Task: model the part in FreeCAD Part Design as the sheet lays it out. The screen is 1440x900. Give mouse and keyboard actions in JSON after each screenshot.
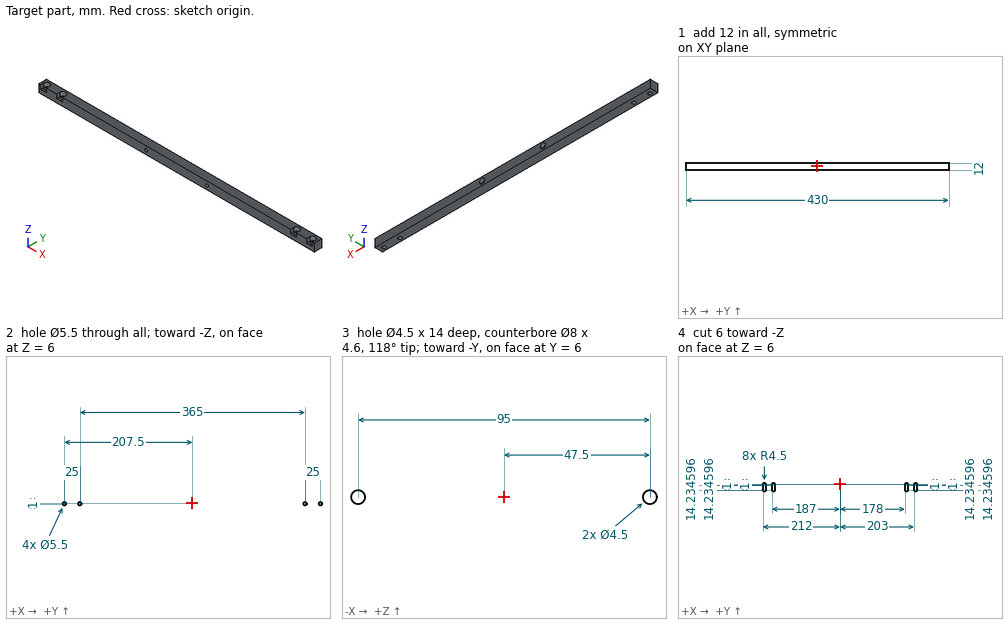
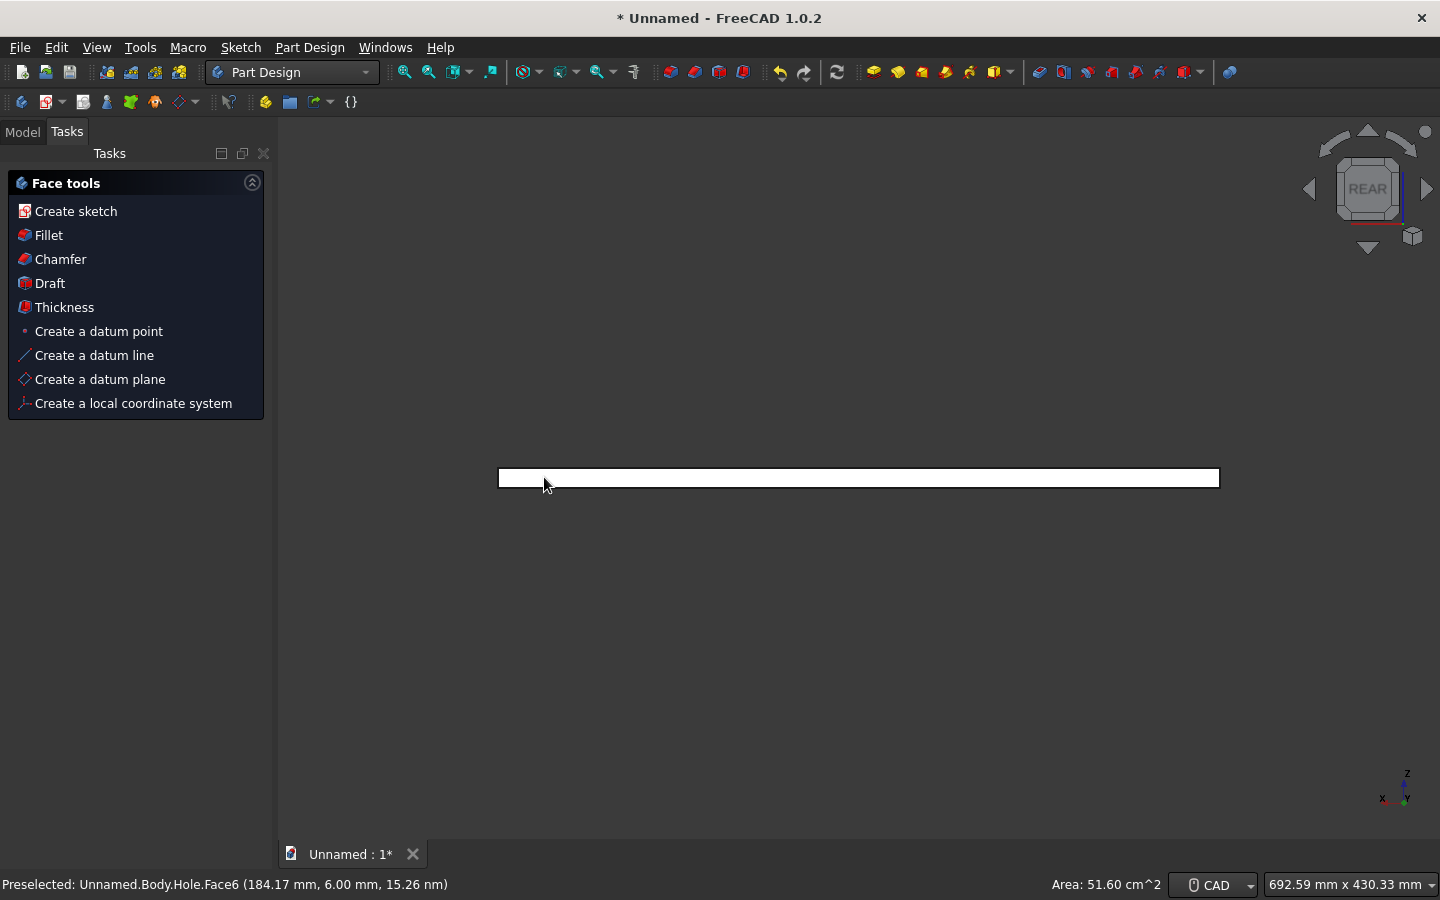
{"action": "left_click", "coordinate": [46, 102]}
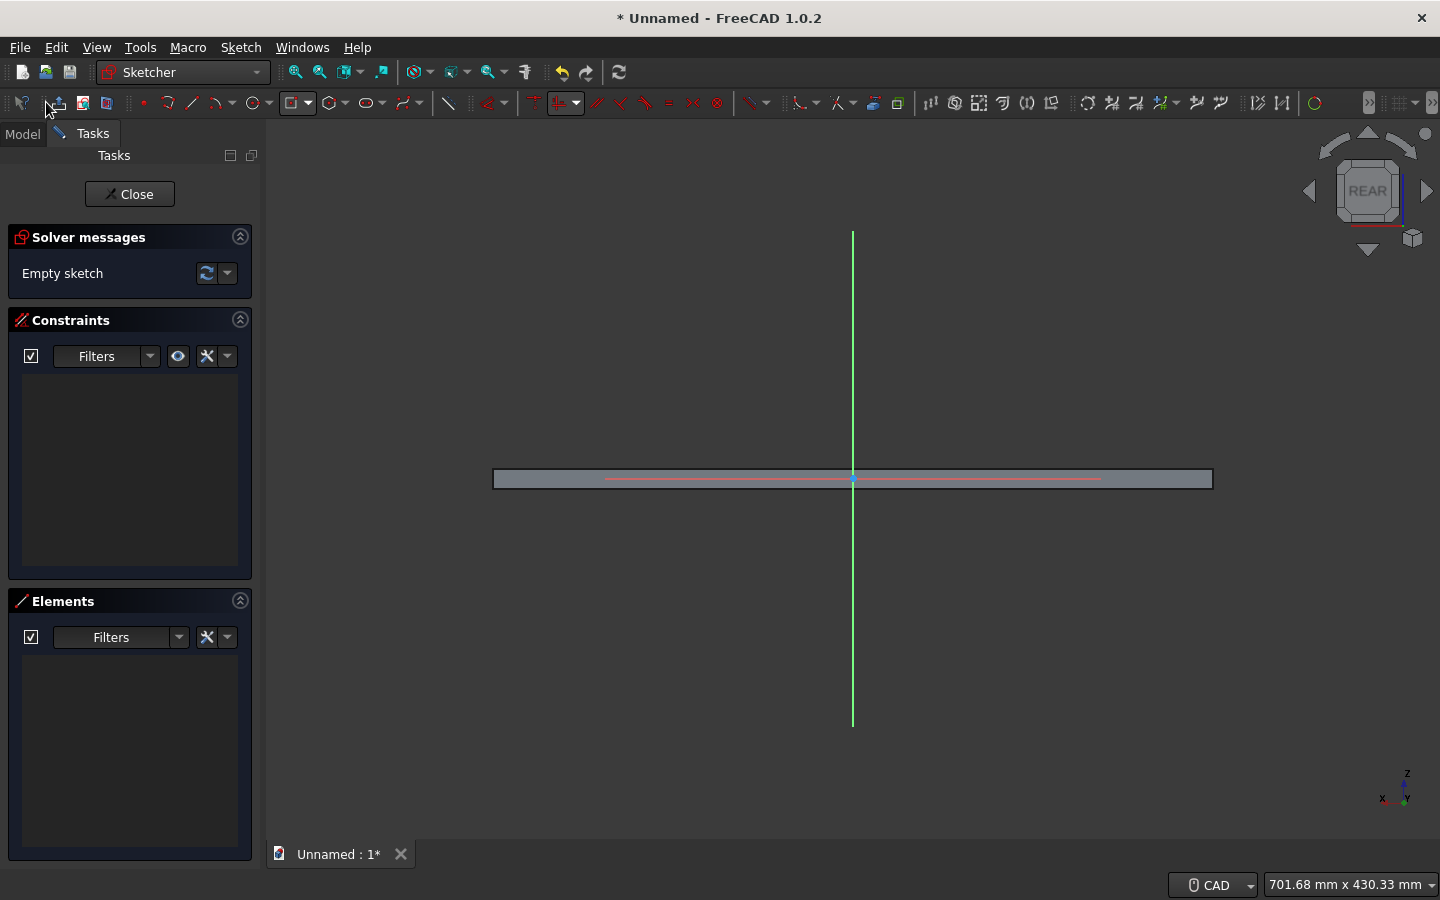
{"action": "scroll", "coordinate": [875, 479], "scroll_direction": "up", "scroll_amount": 7}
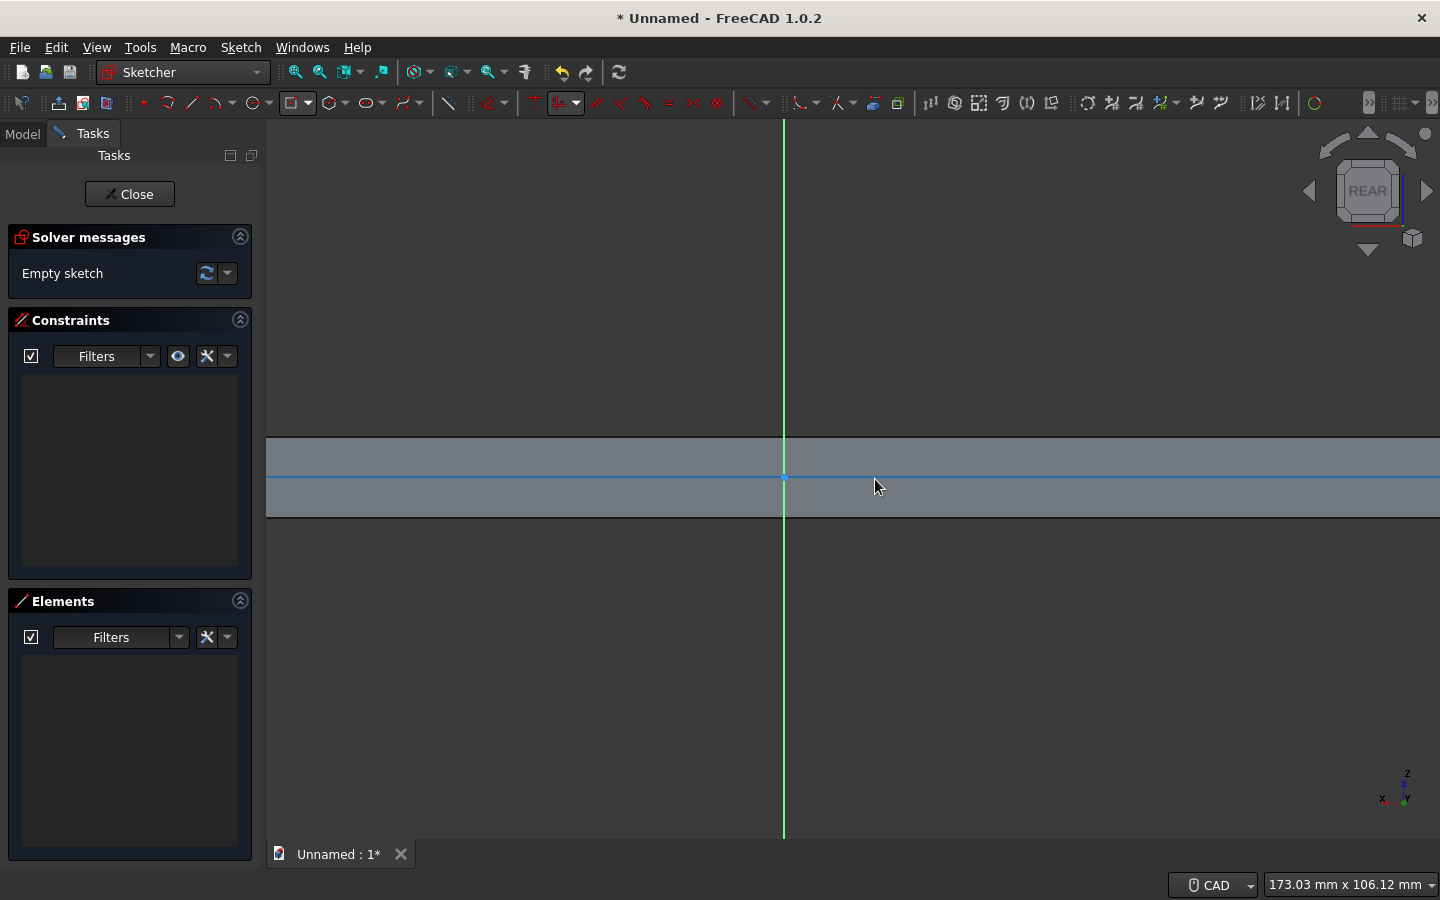
{"action": "left_click", "coordinate": [254, 104]}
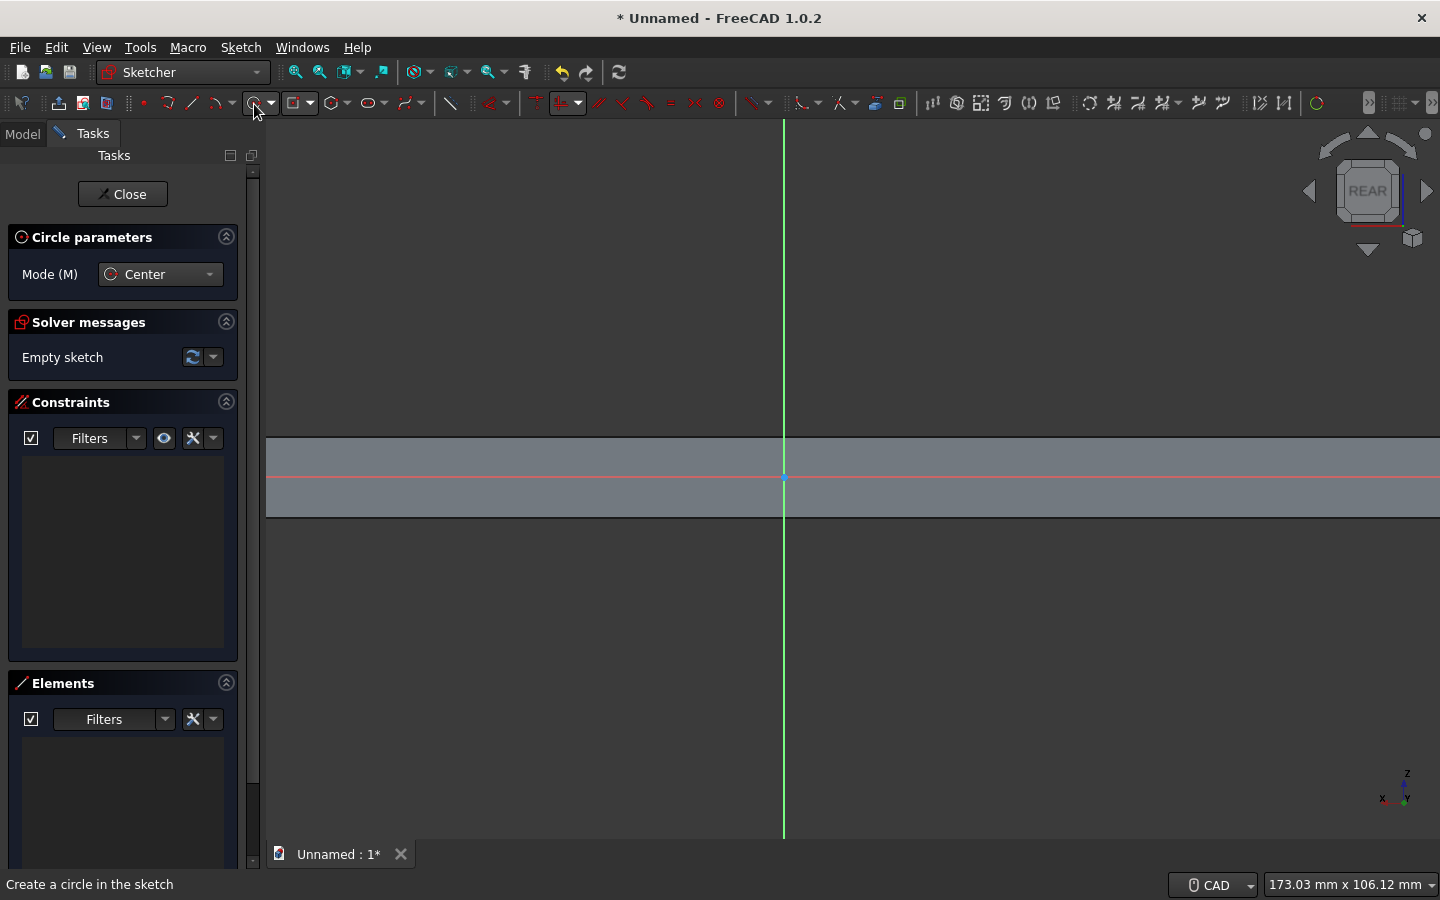
{"action": "scroll", "coordinate": [1106, 477], "scroll_direction": "up", "scroll_amount": 2}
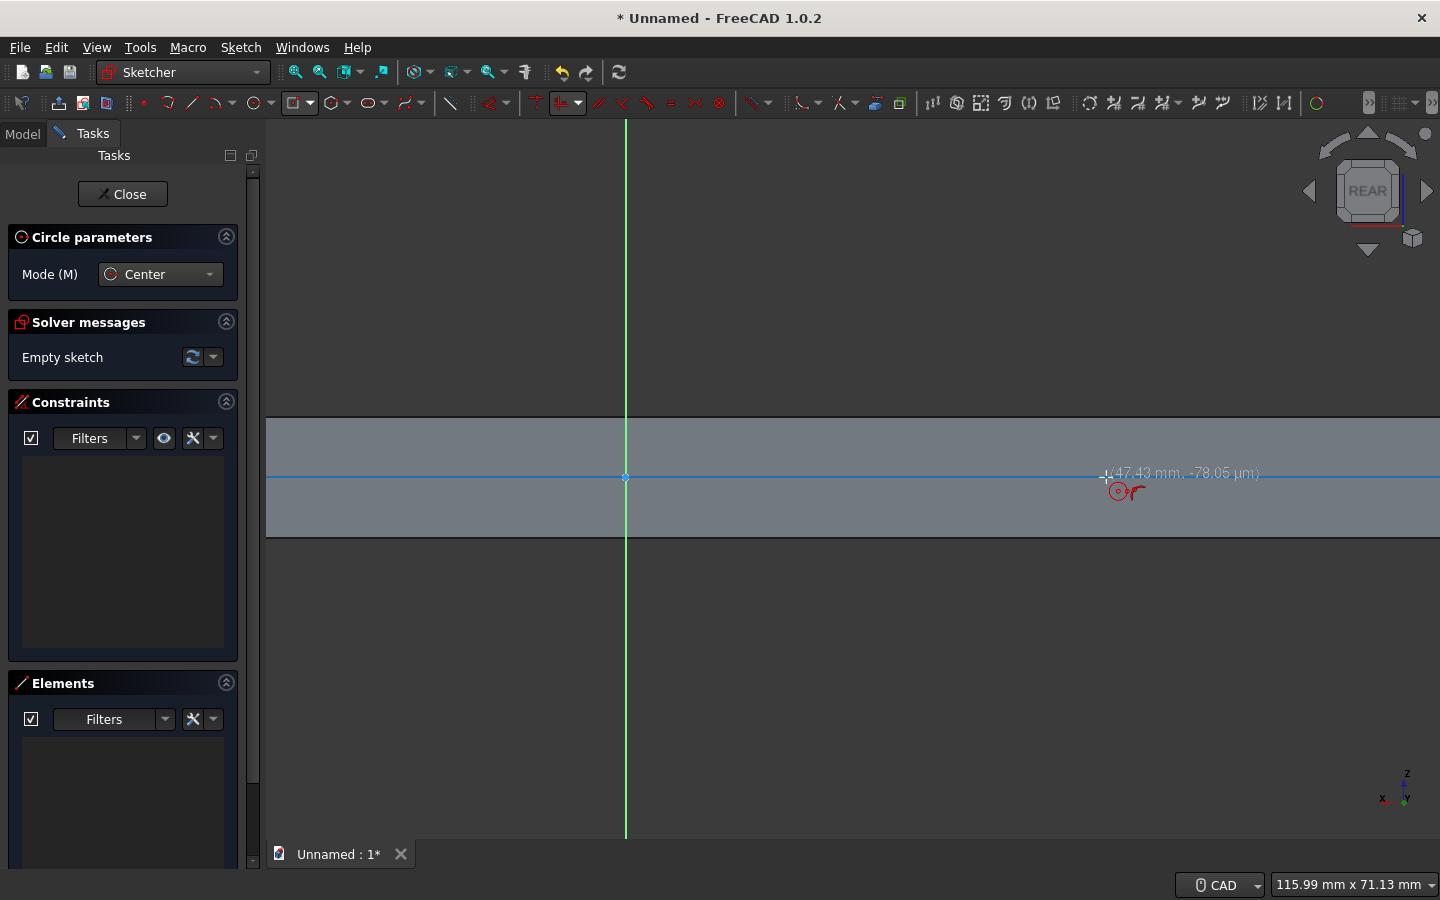
{"action": "left_click", "coordinate": [1106, 477]}
{"action": "mouse_move", "coordinate": [1122, 461]}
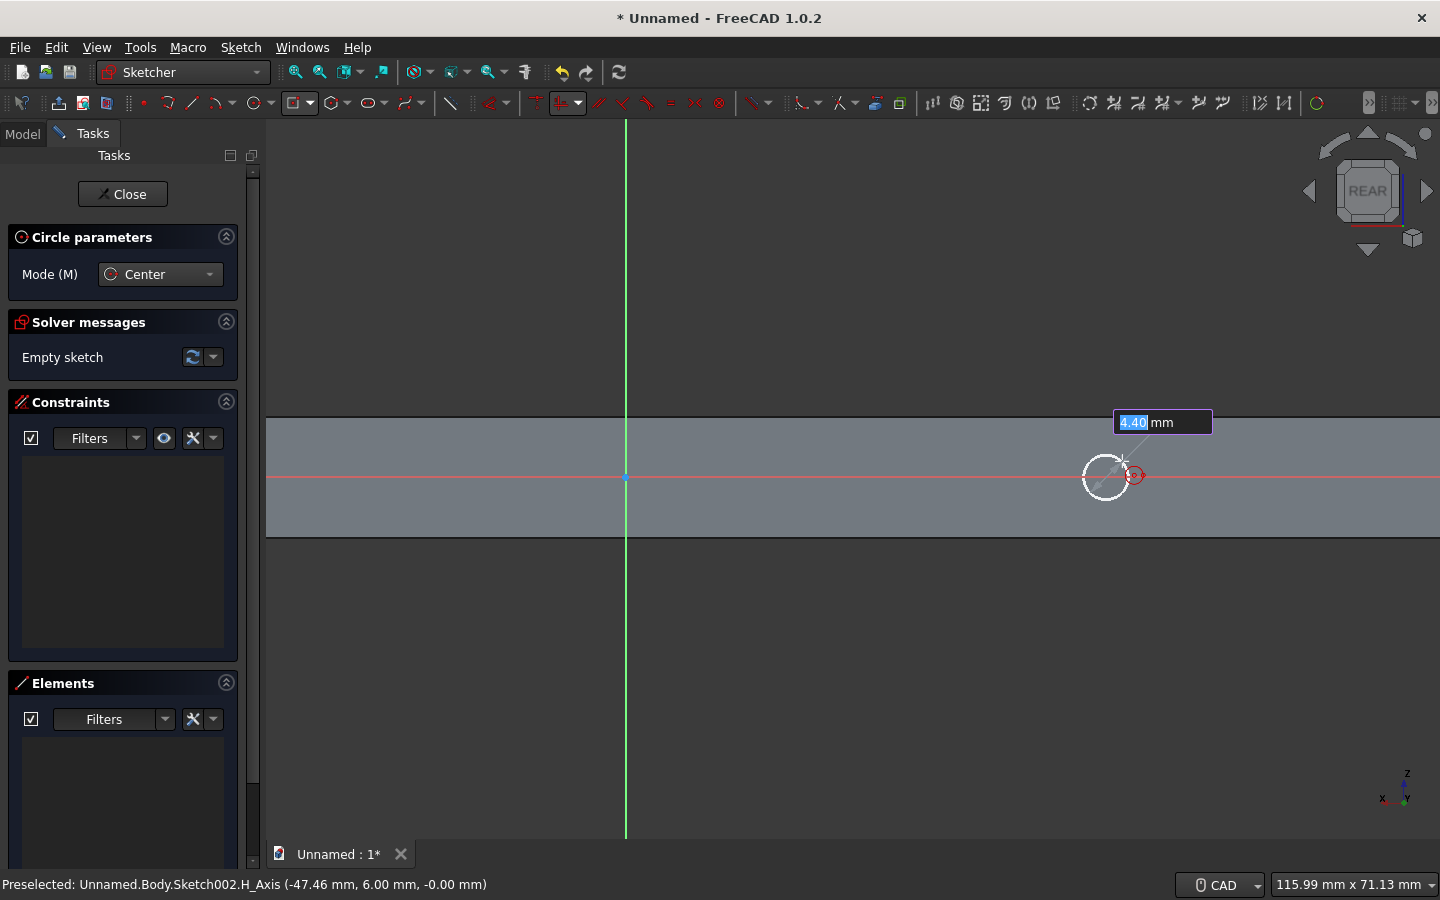
{"action": "type", "text": "4.5"}
{"action": "key", "text": "Return"}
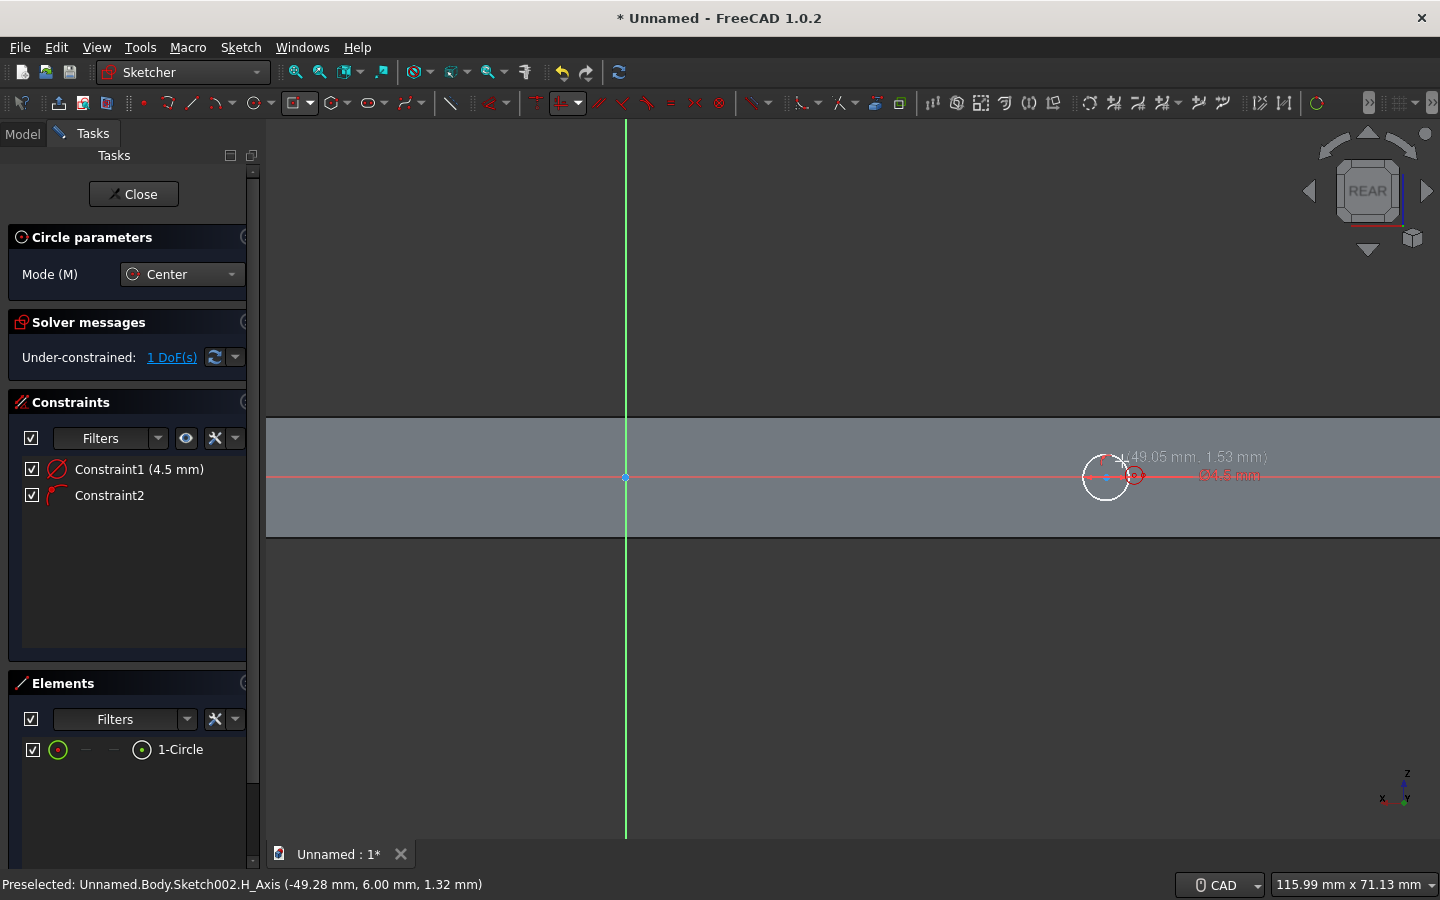
{"action": "scroll", "coordinate": [1108, 482], "scroll_direction": "down", "scroll_amount": 2}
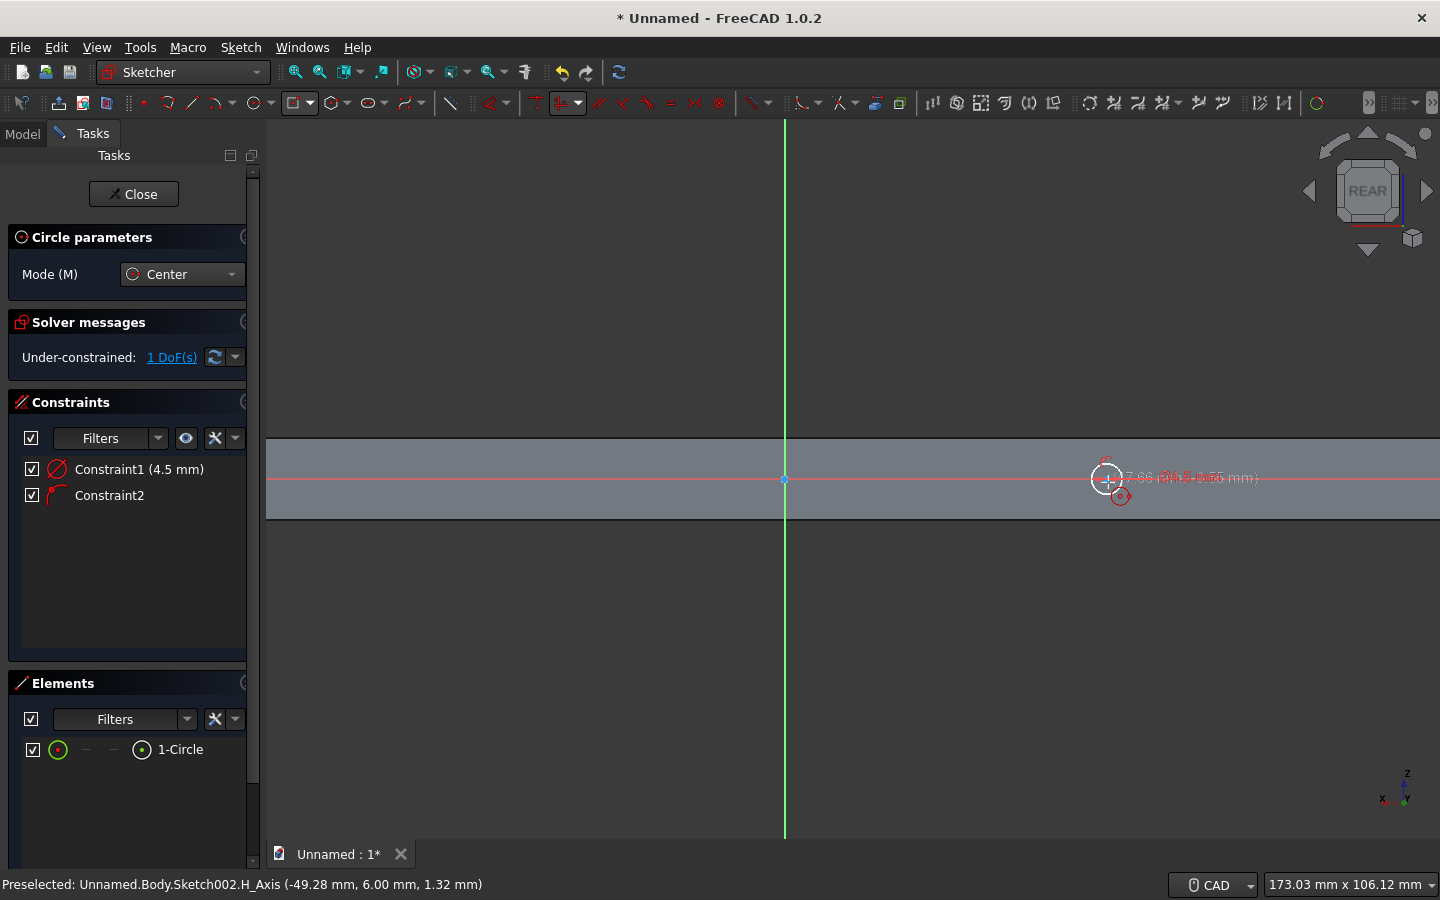
{"action": "scroll", "coordinate": [463, 479], "scroll_direction": "up", "scroll_amount": 2}